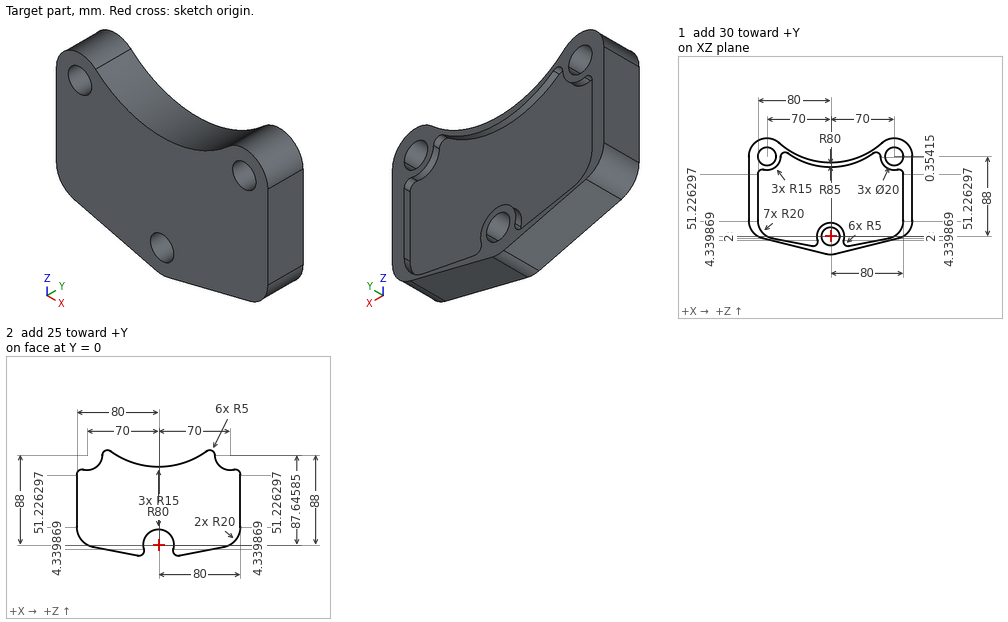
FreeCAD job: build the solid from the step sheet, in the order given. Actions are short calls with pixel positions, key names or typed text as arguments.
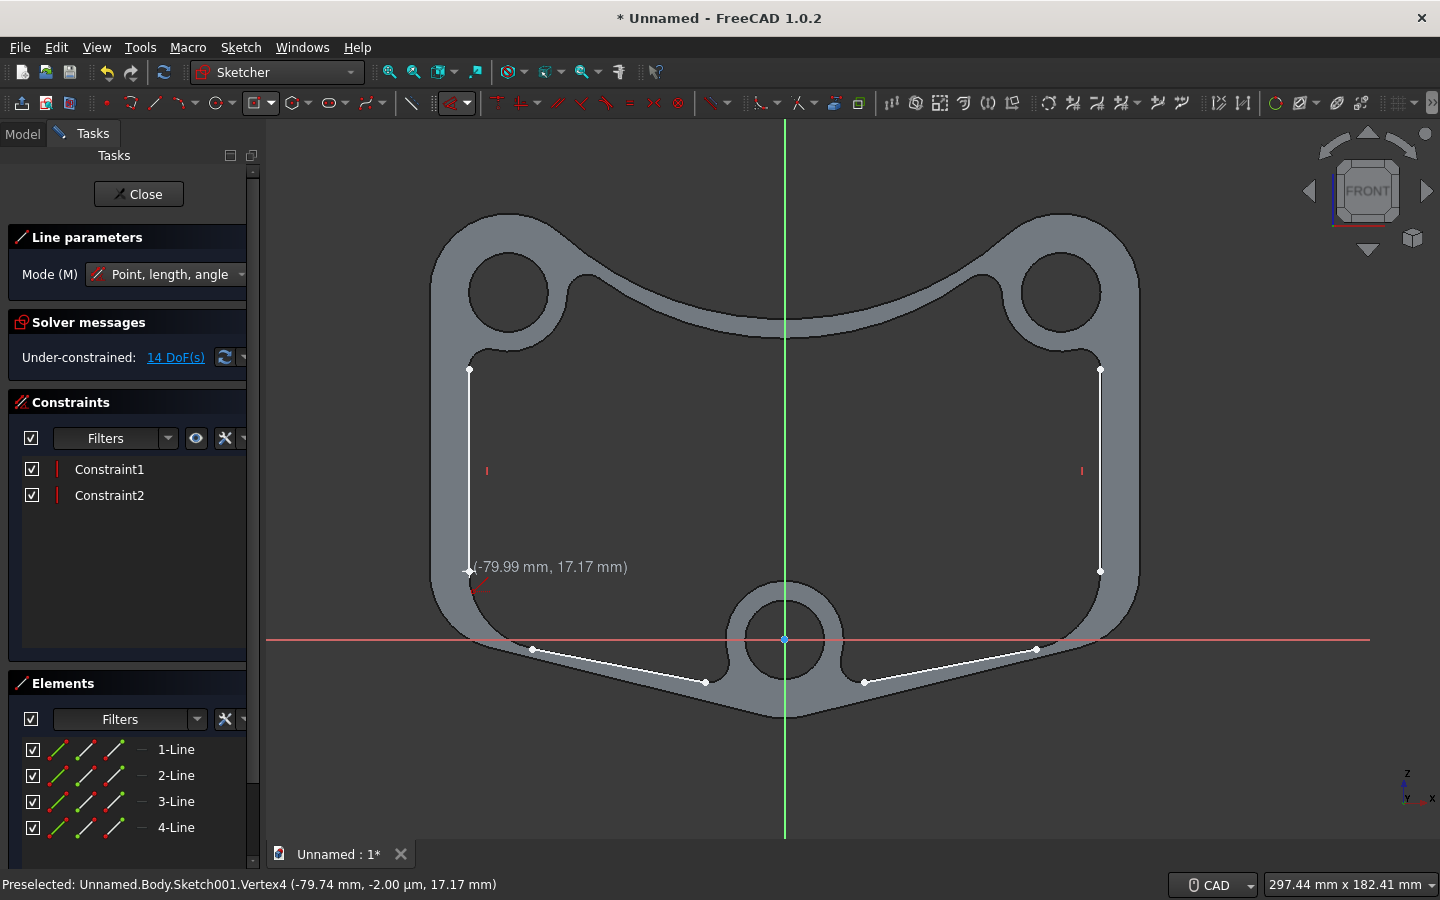
click(180, 104)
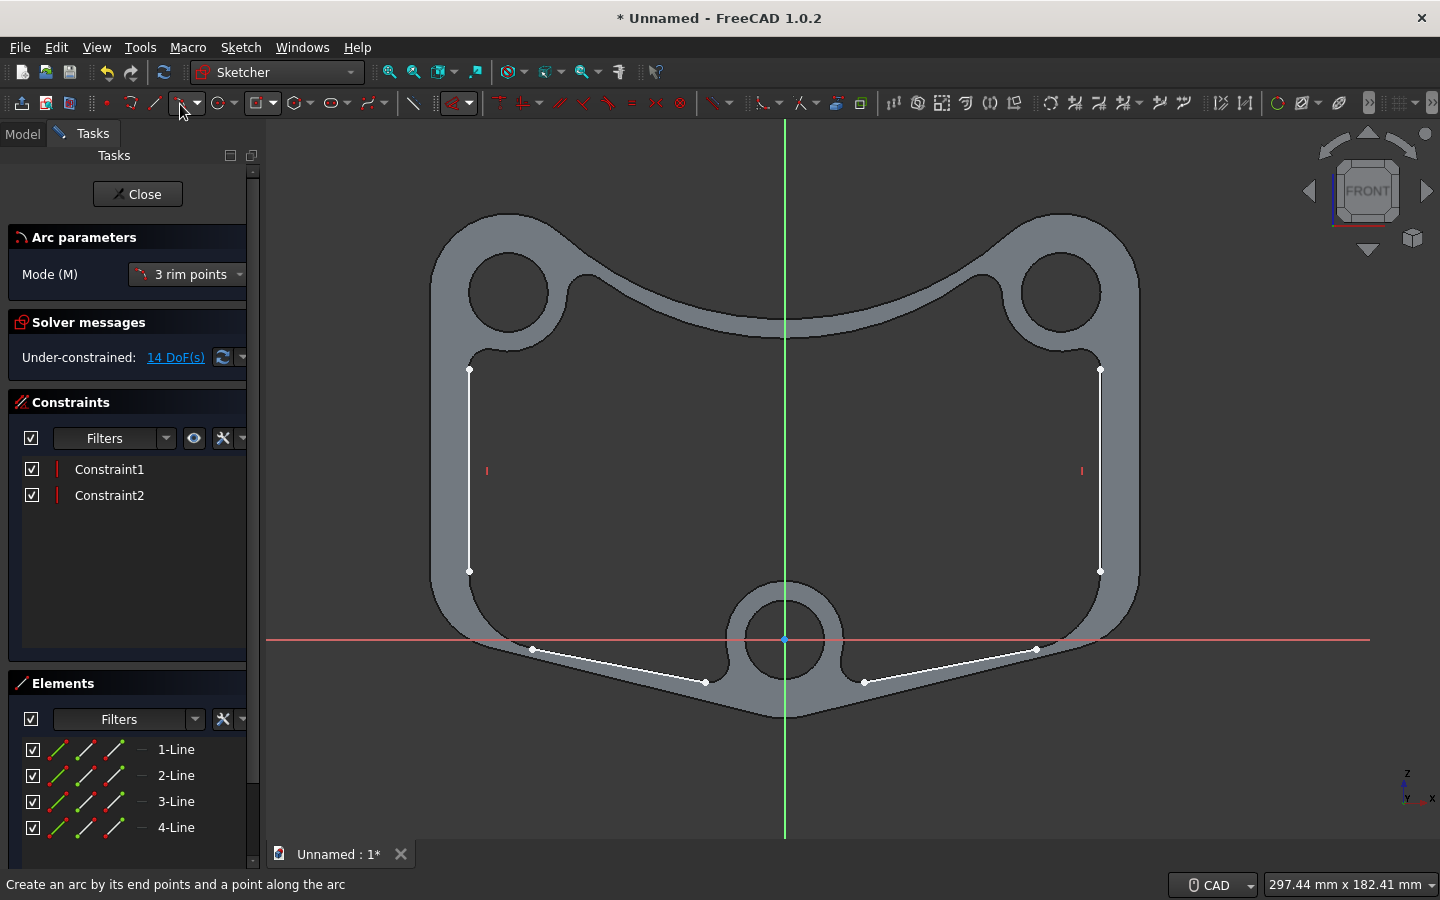
click(706, 683)
click(728, 657)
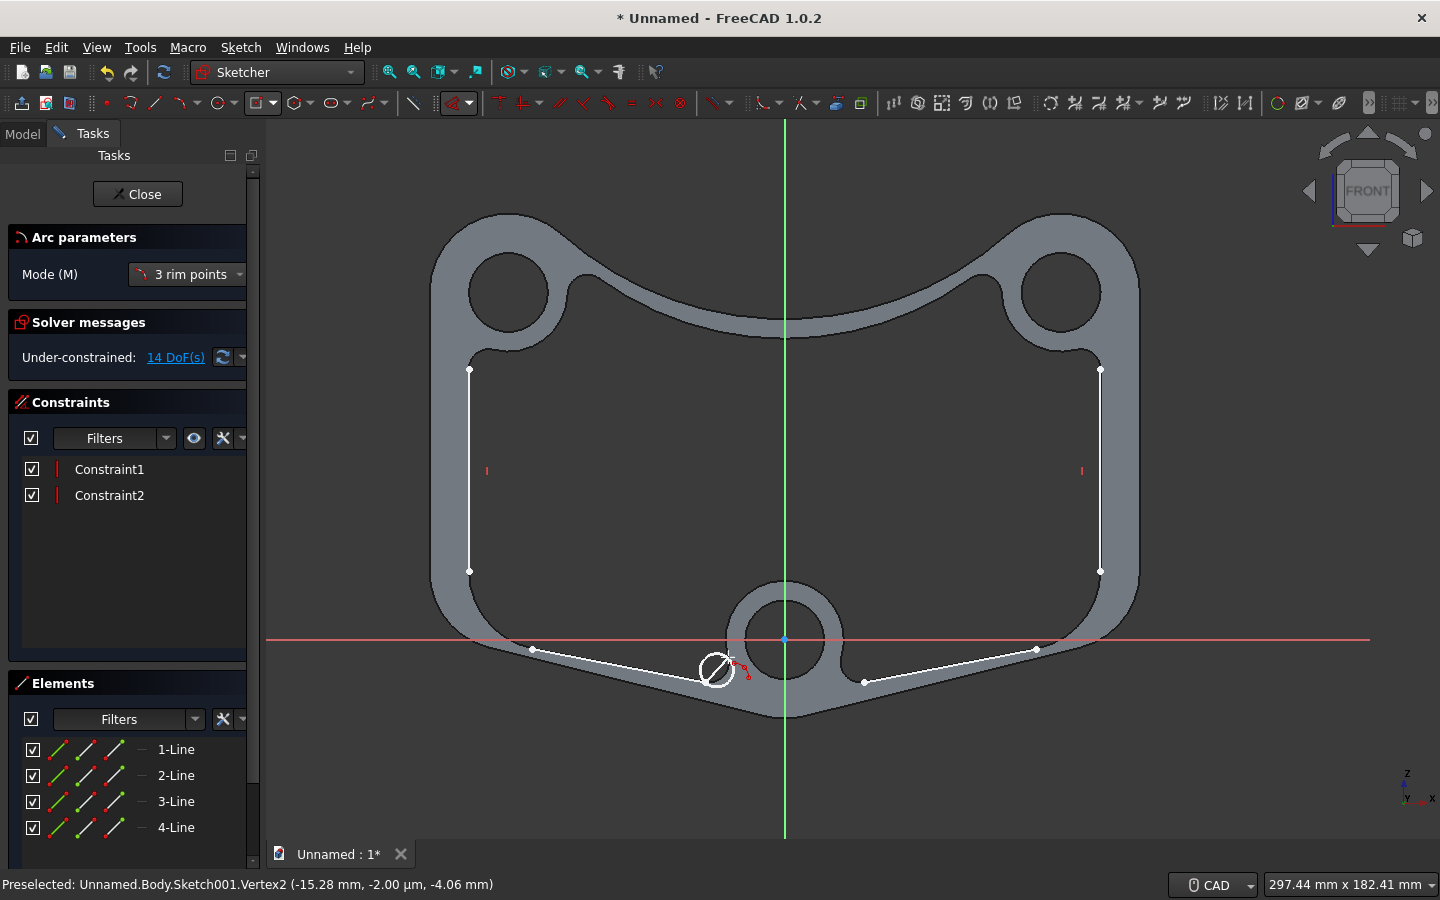
scroll(724, 676, up, 3)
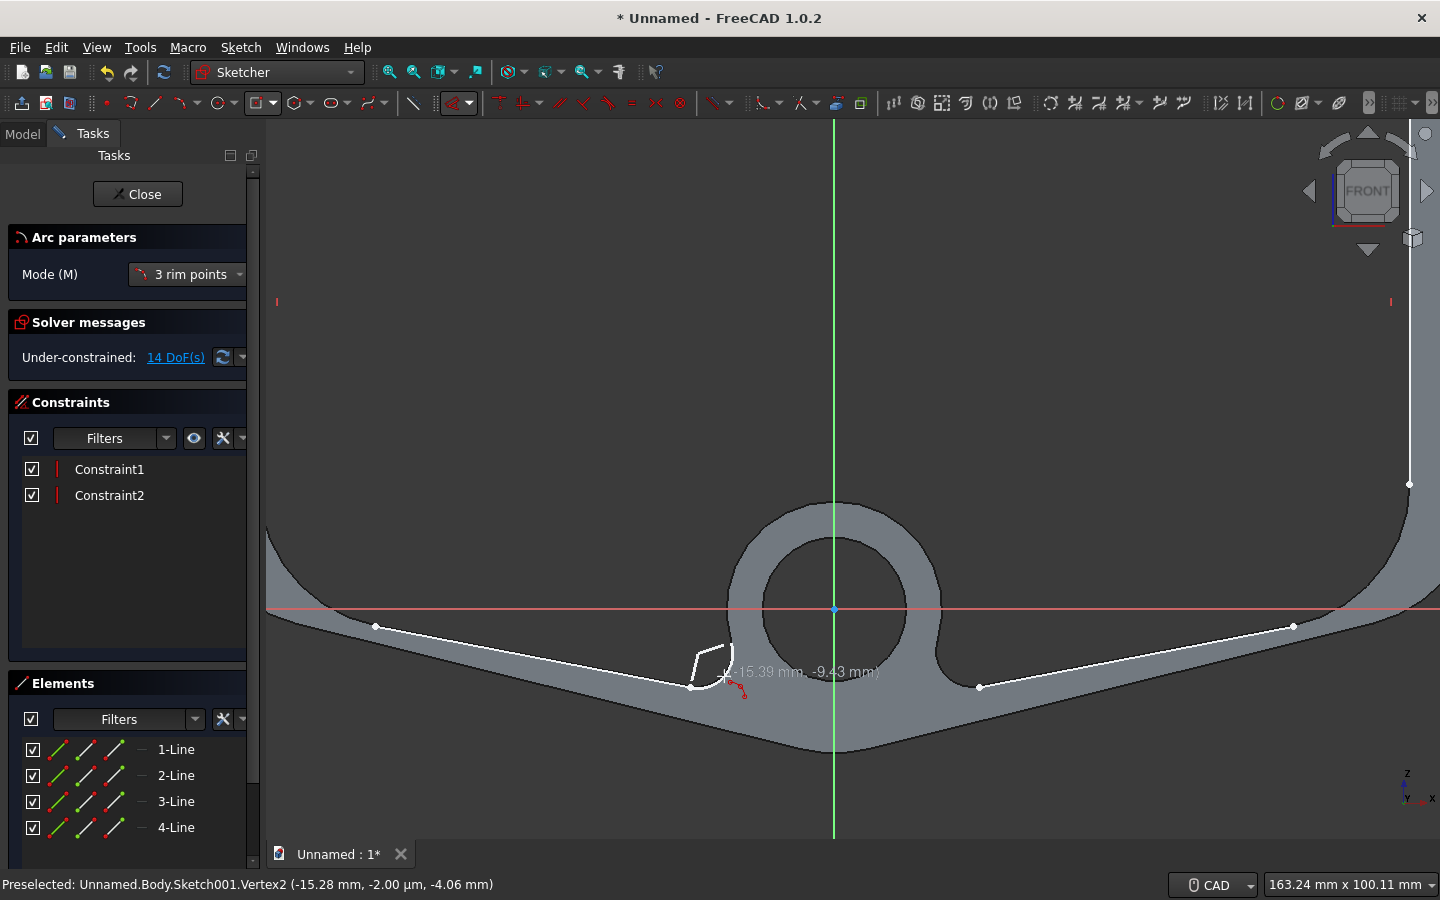
click(723, 675)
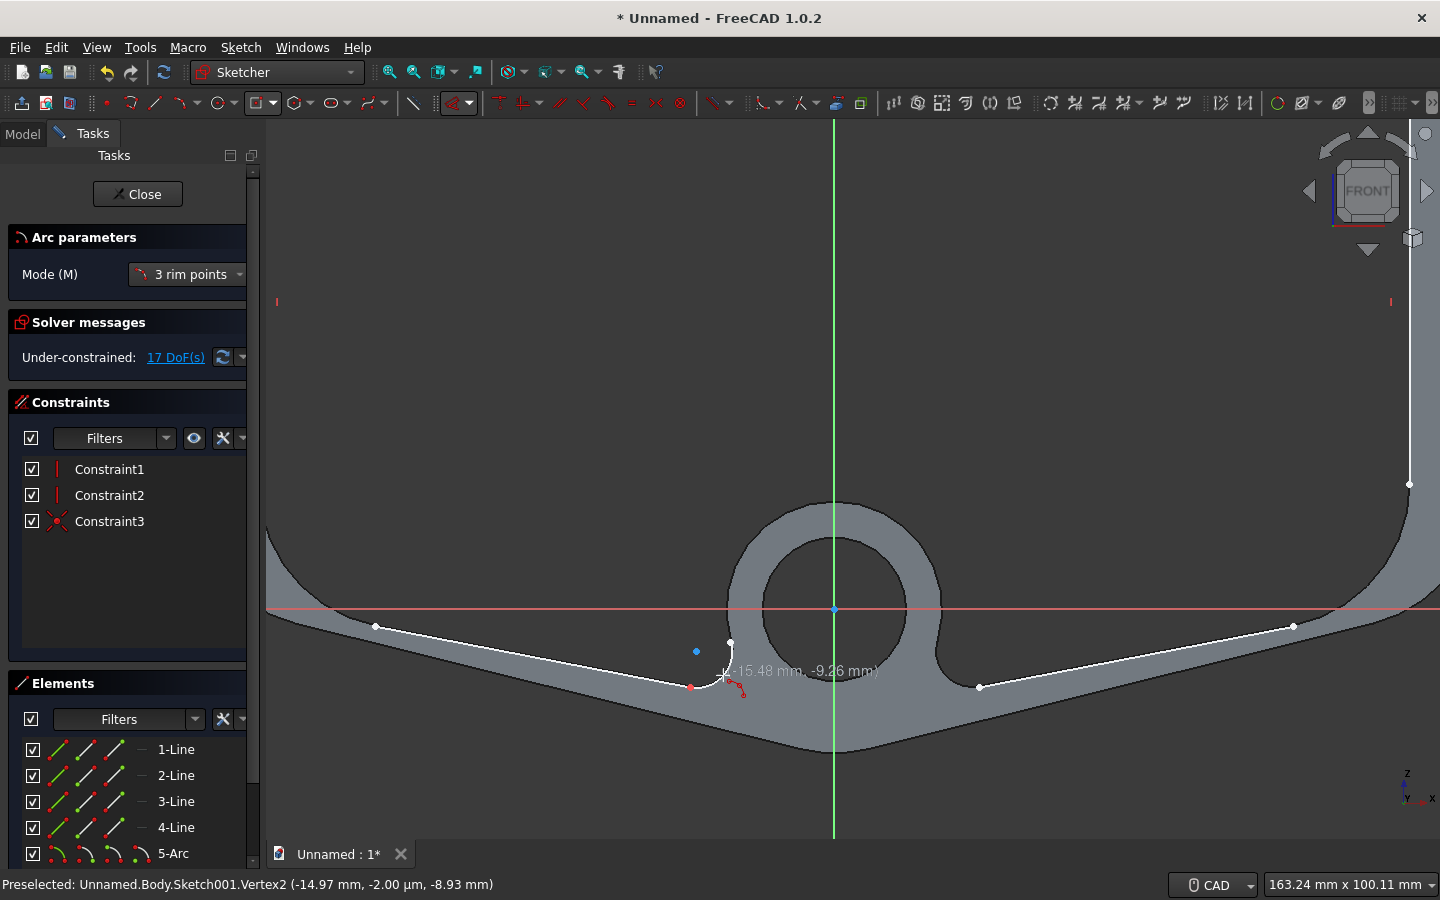
click(731, 643)
click(938, 641)
click(874, 509)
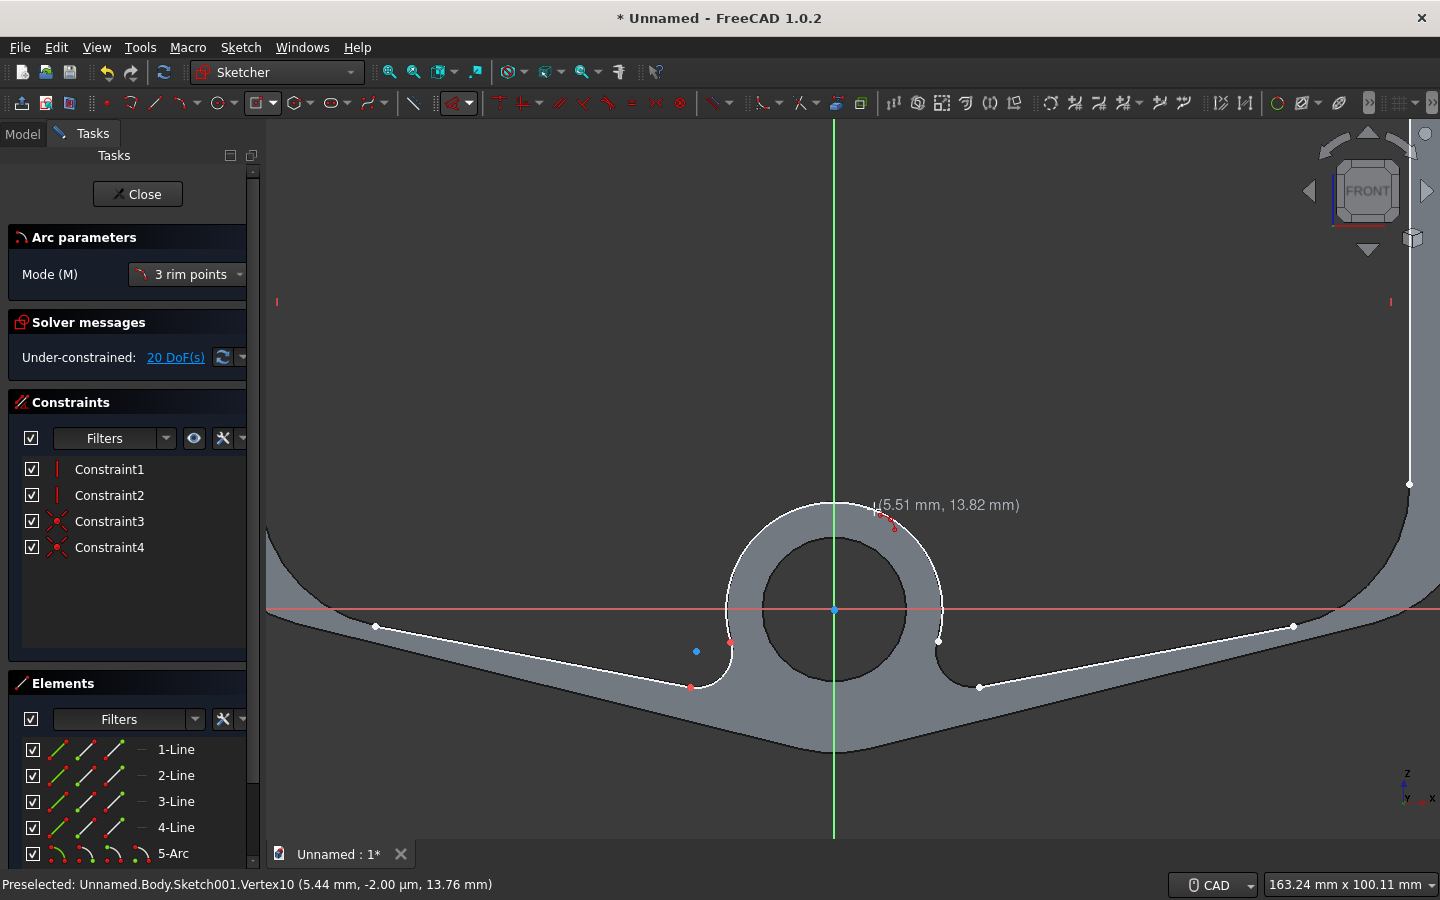
click(938, 642)
click(979, 688)
click(945, 675)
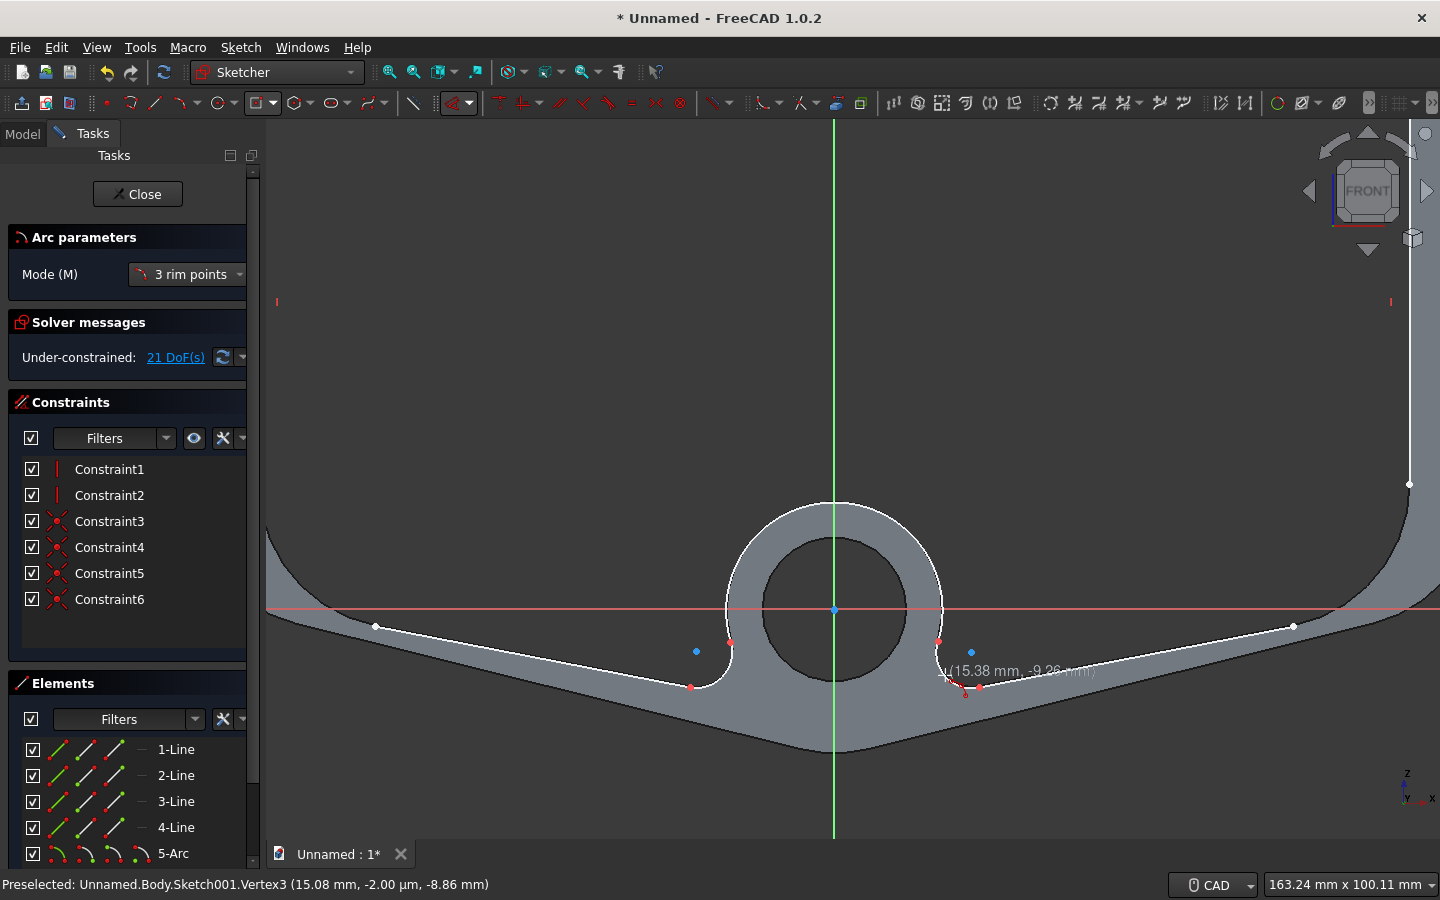
scroll(724, 676, down, 3)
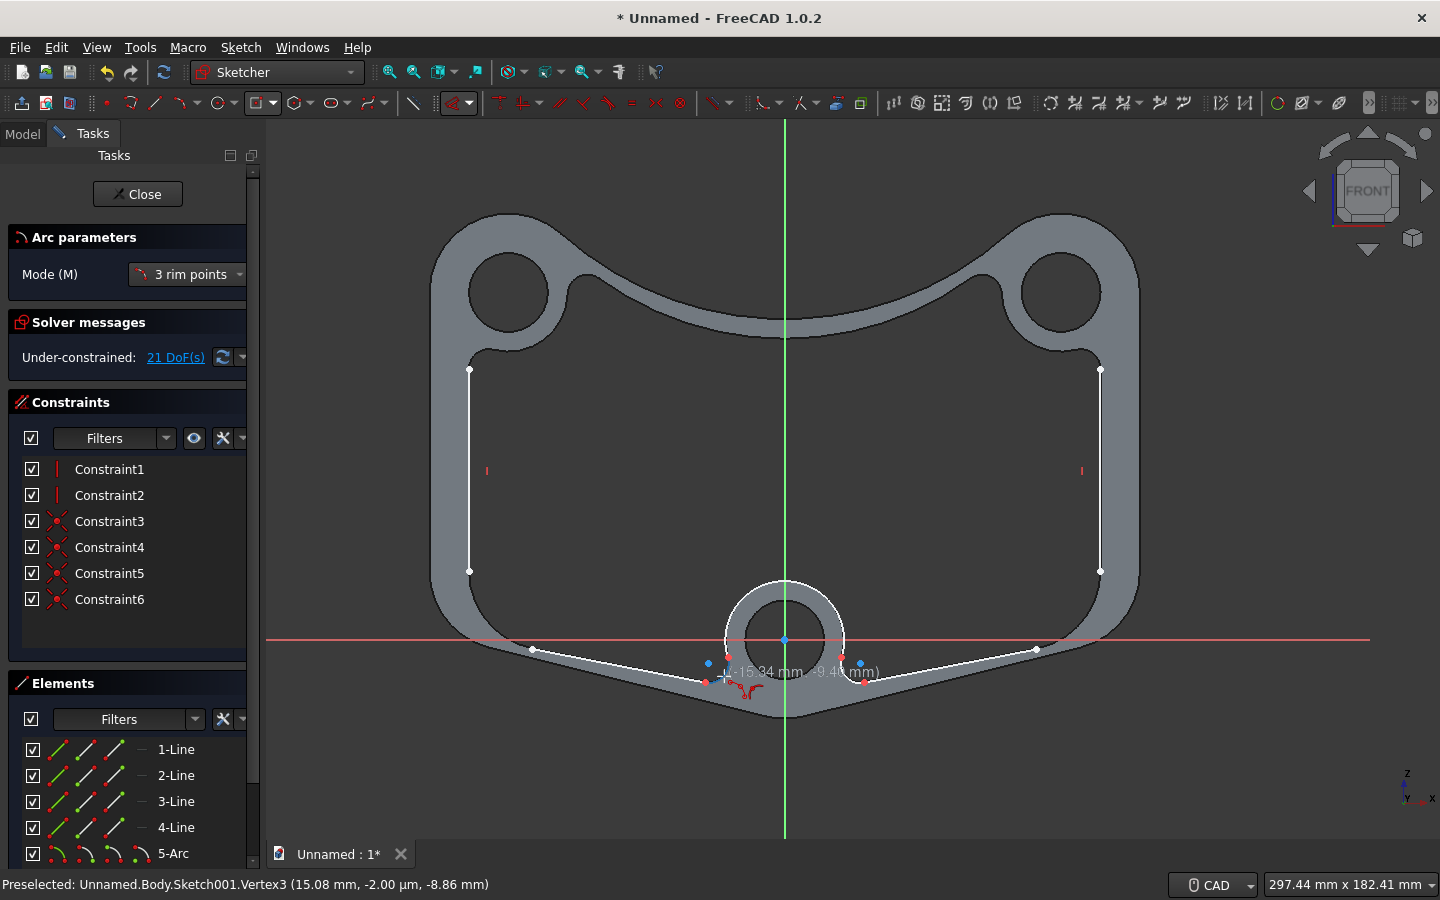
scroll(1037, 649, up, 3)